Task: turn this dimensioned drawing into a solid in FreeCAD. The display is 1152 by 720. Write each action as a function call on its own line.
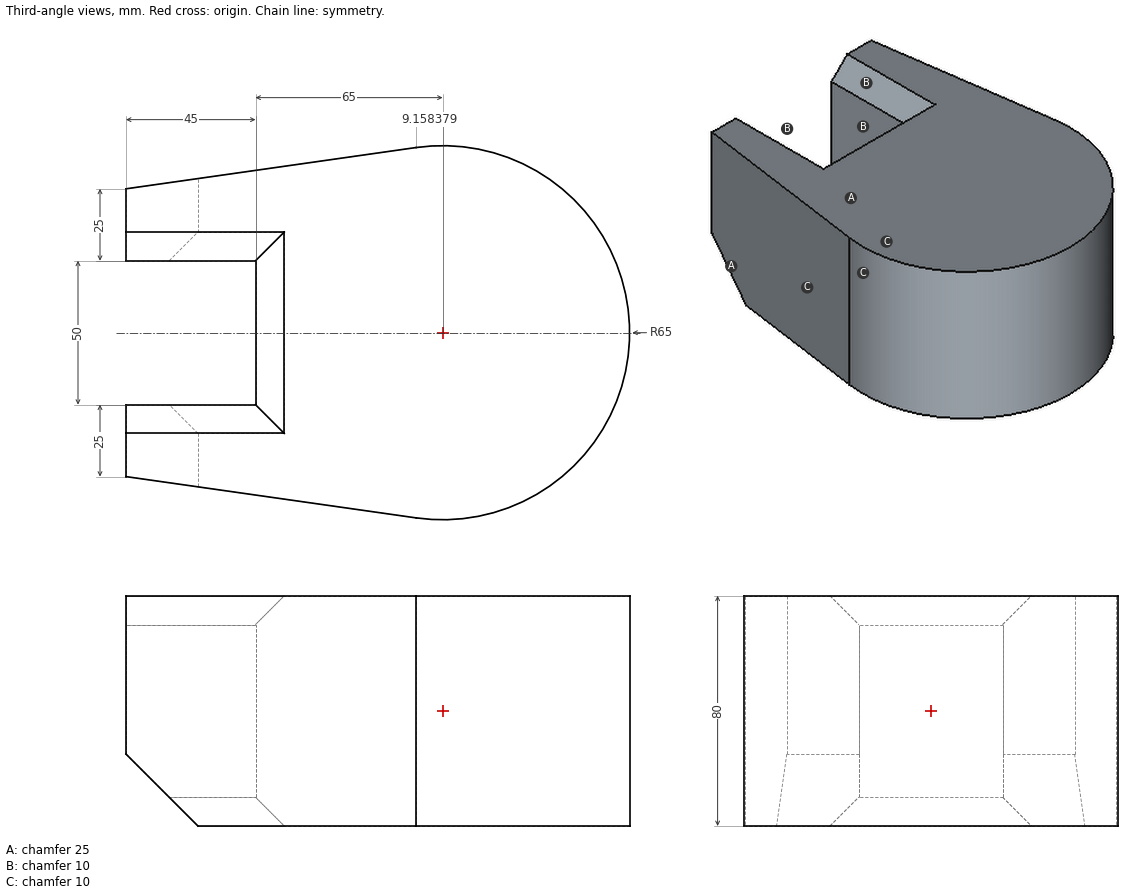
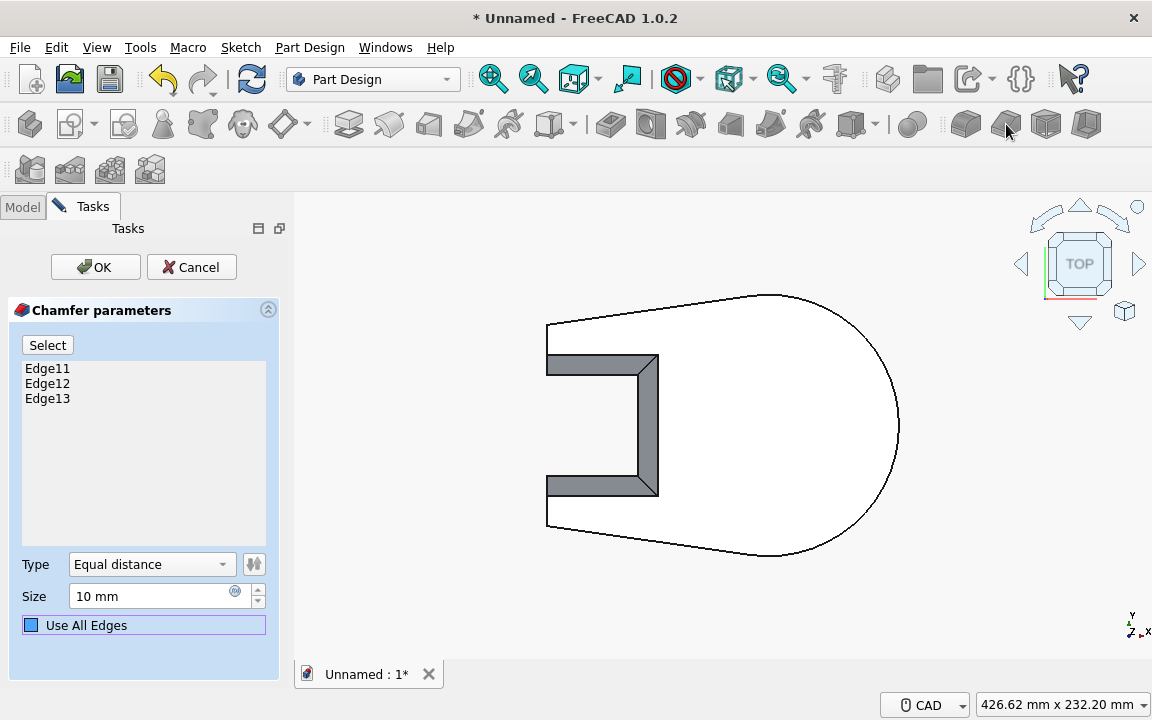
click(96, 267)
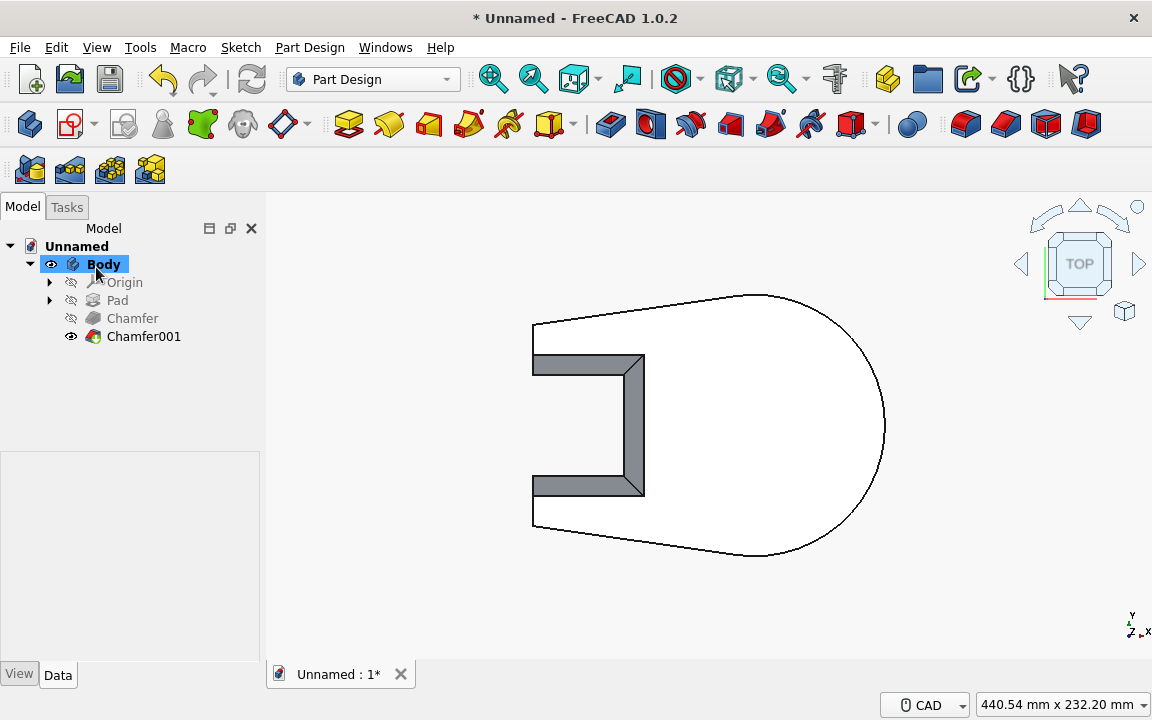
key(0)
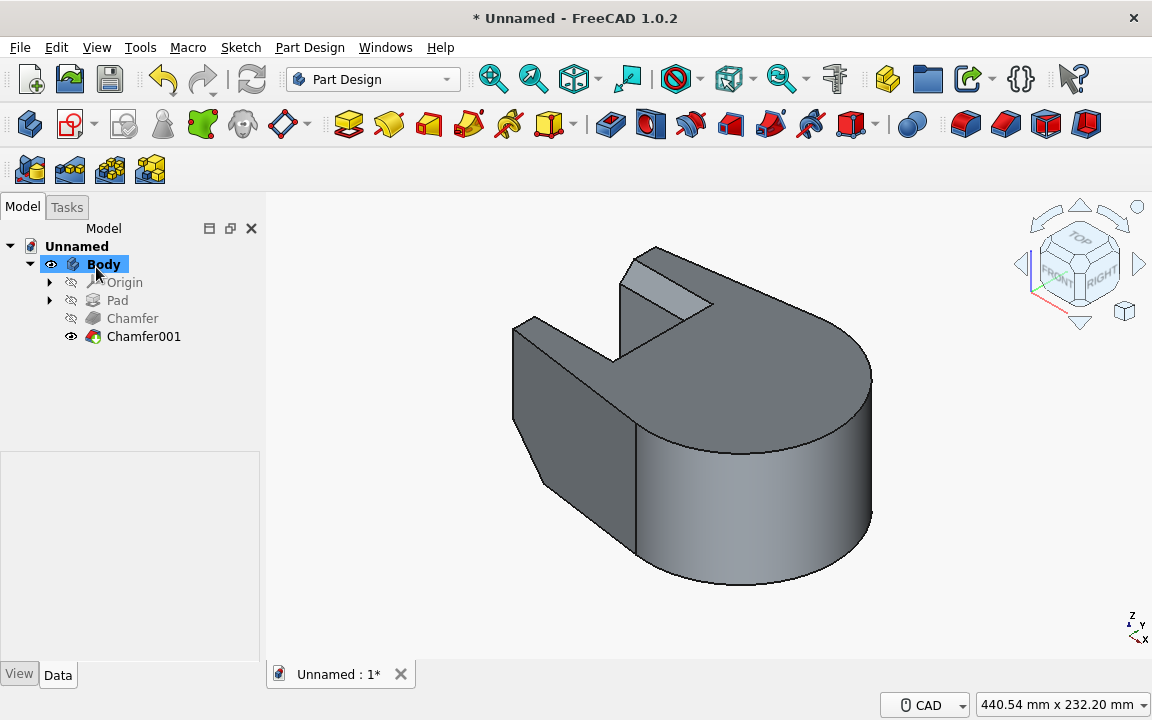
key(2)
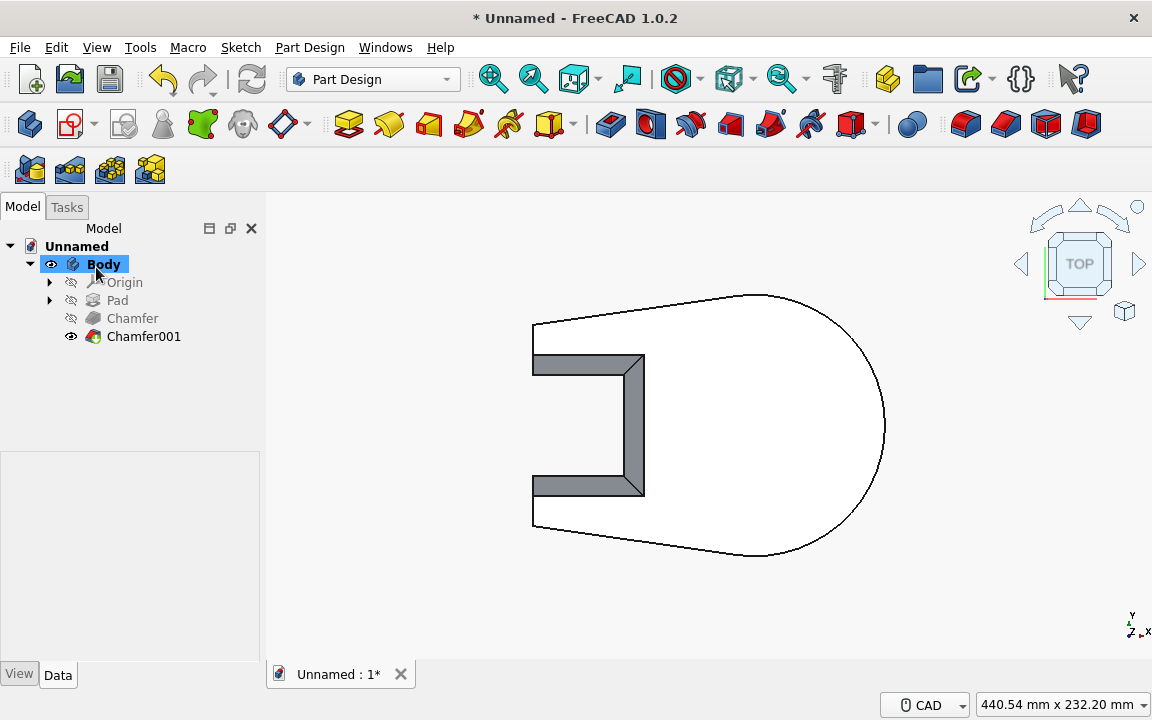
key(1)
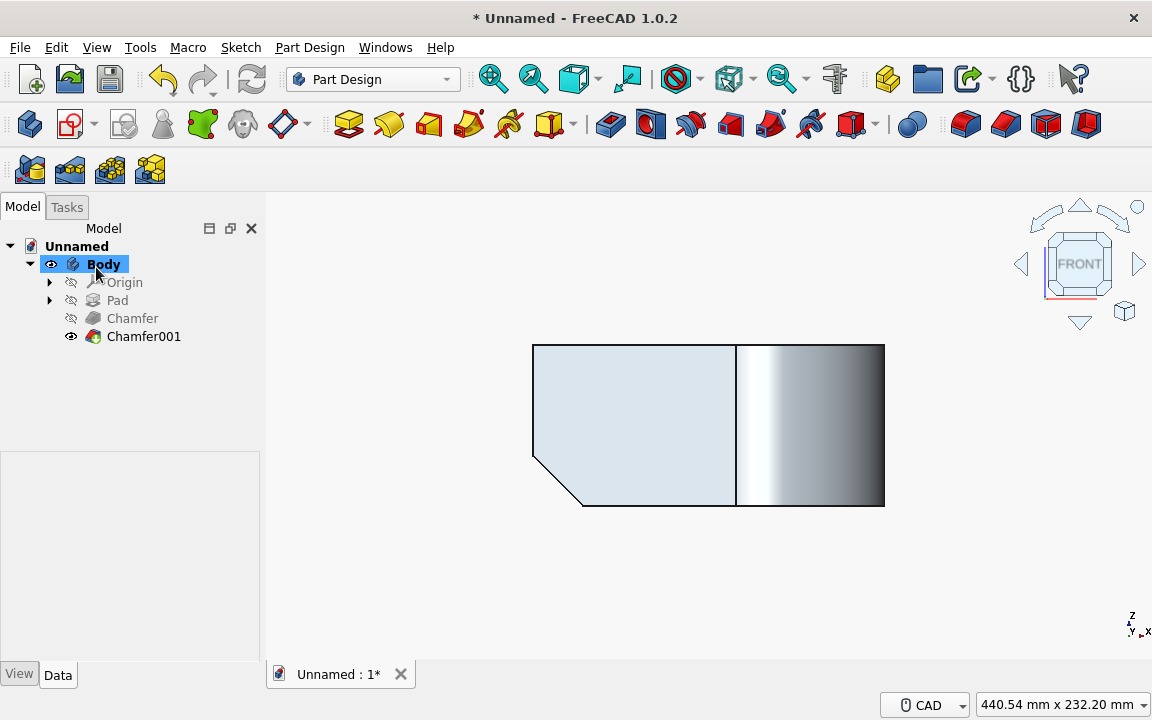
click(494, 80)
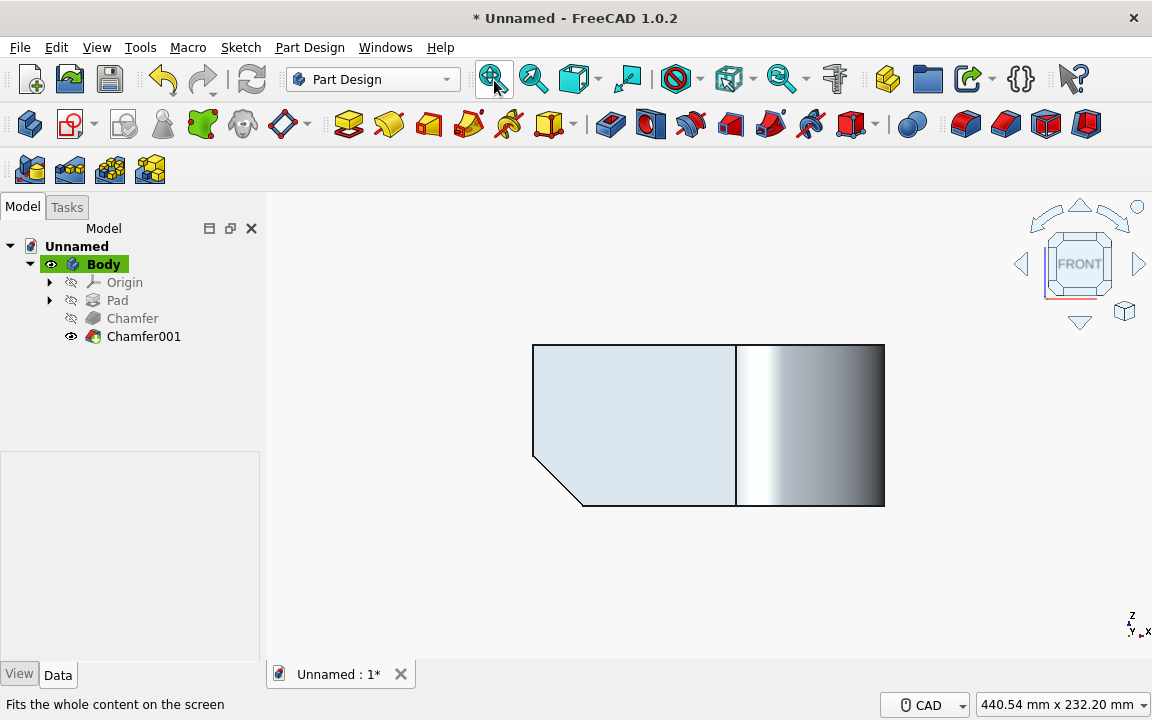
key(3)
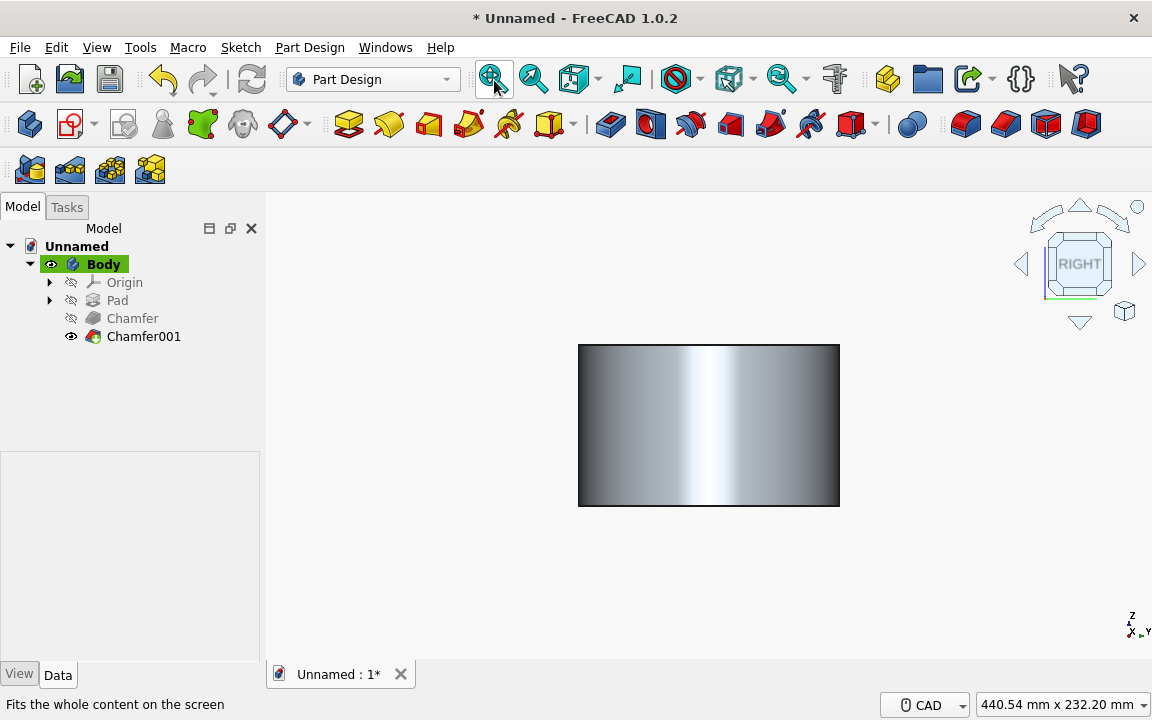
click(494, 80)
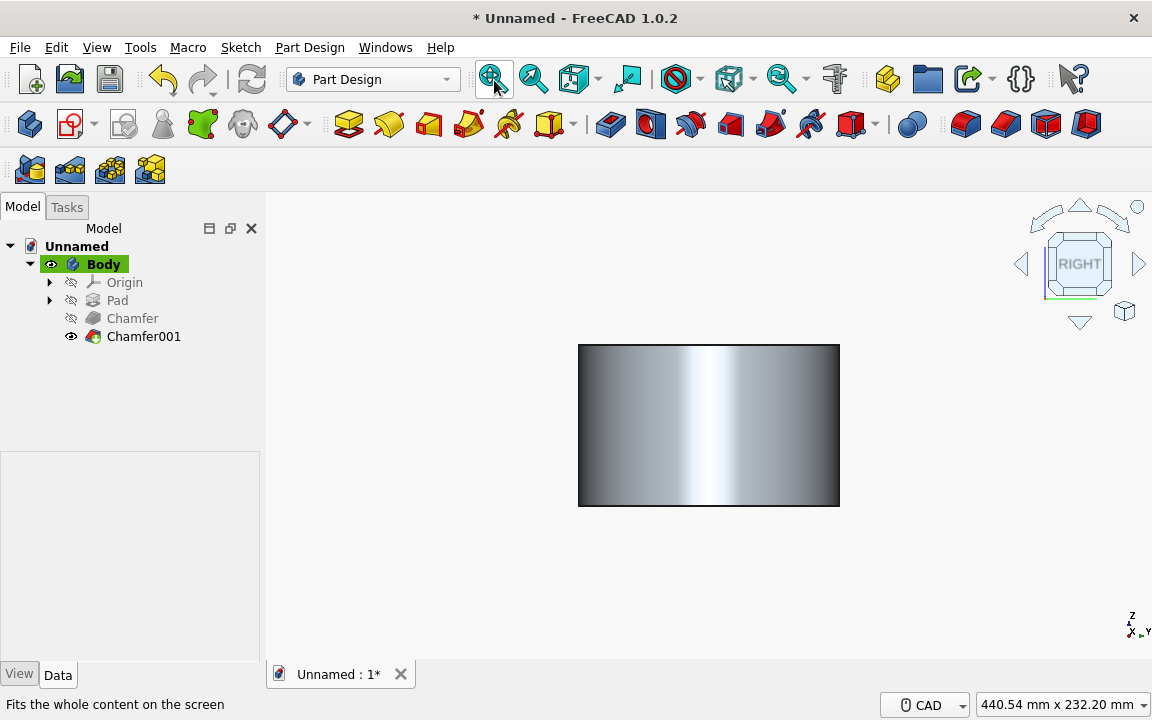
key(5)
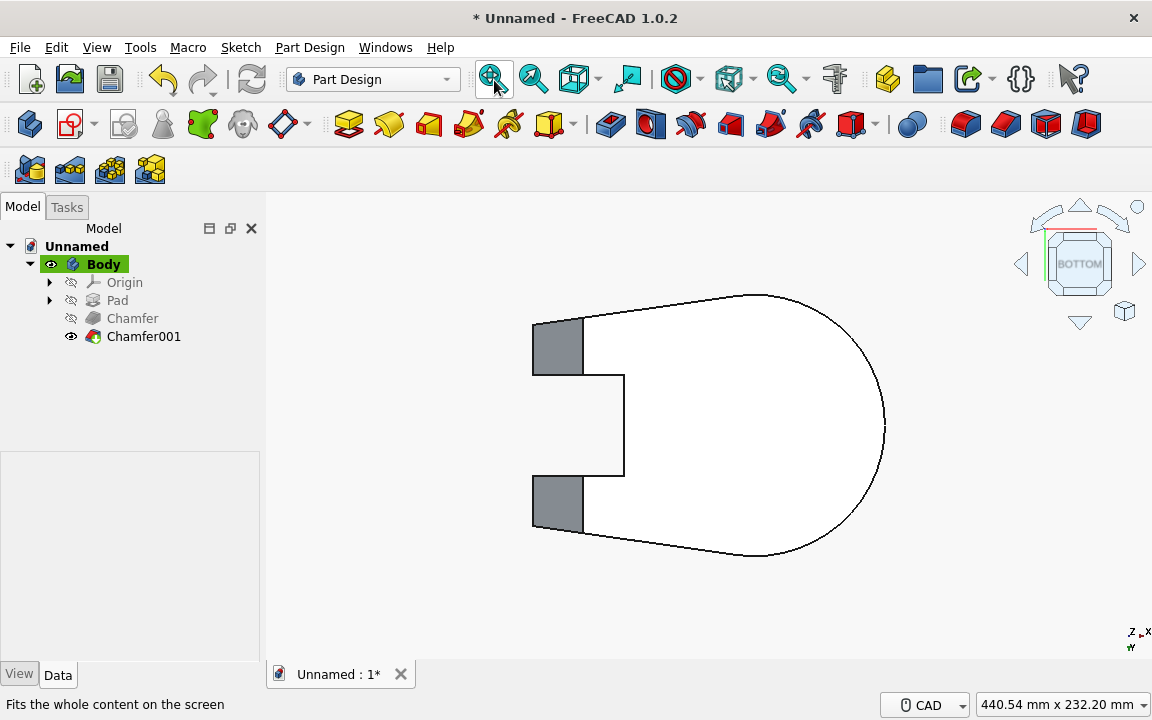
click(603, 475)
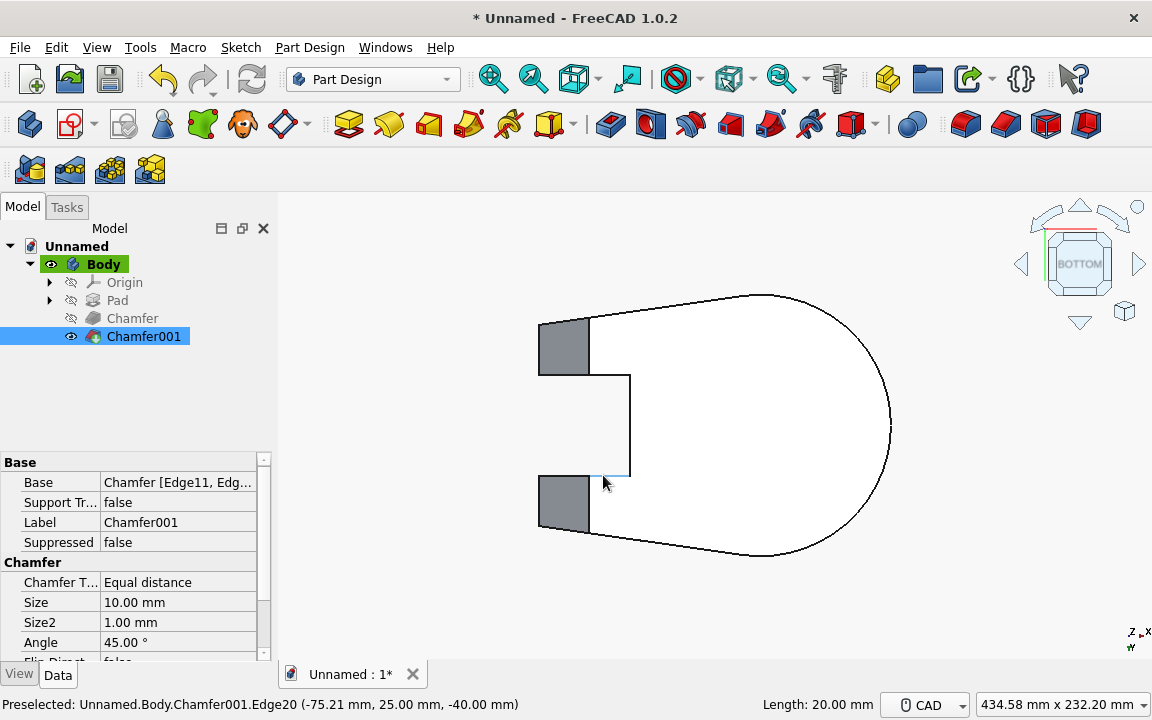
click(609, 374, ctrl)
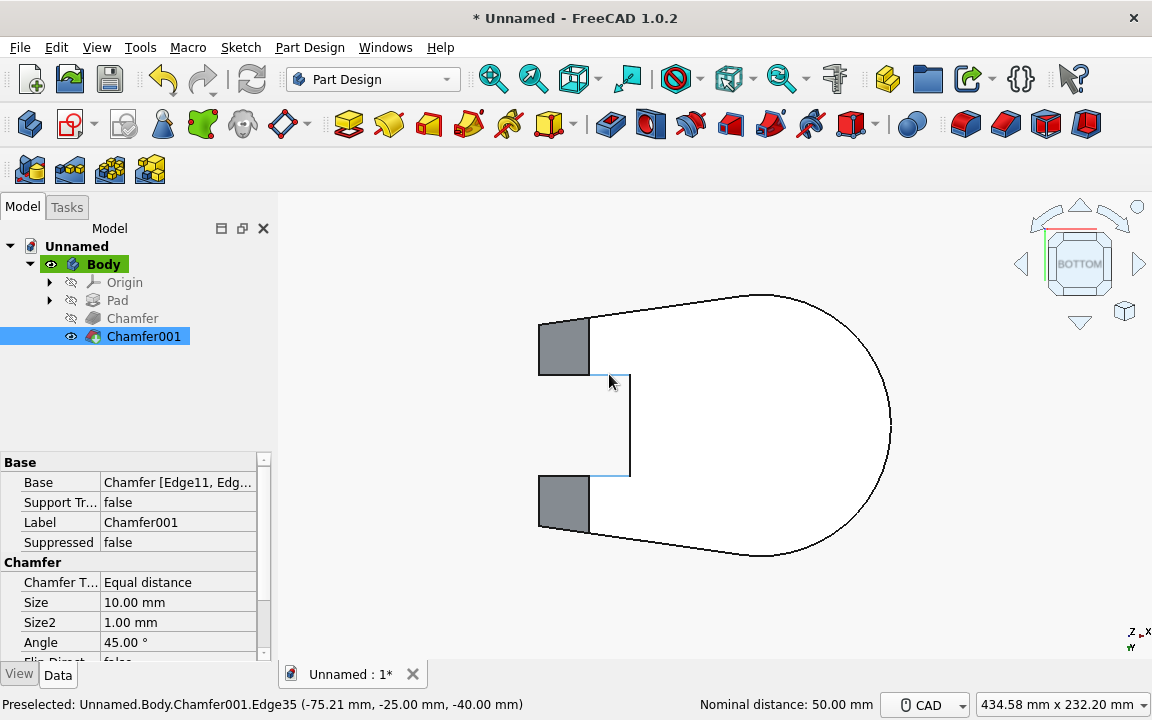
click(630, 424, ctrl)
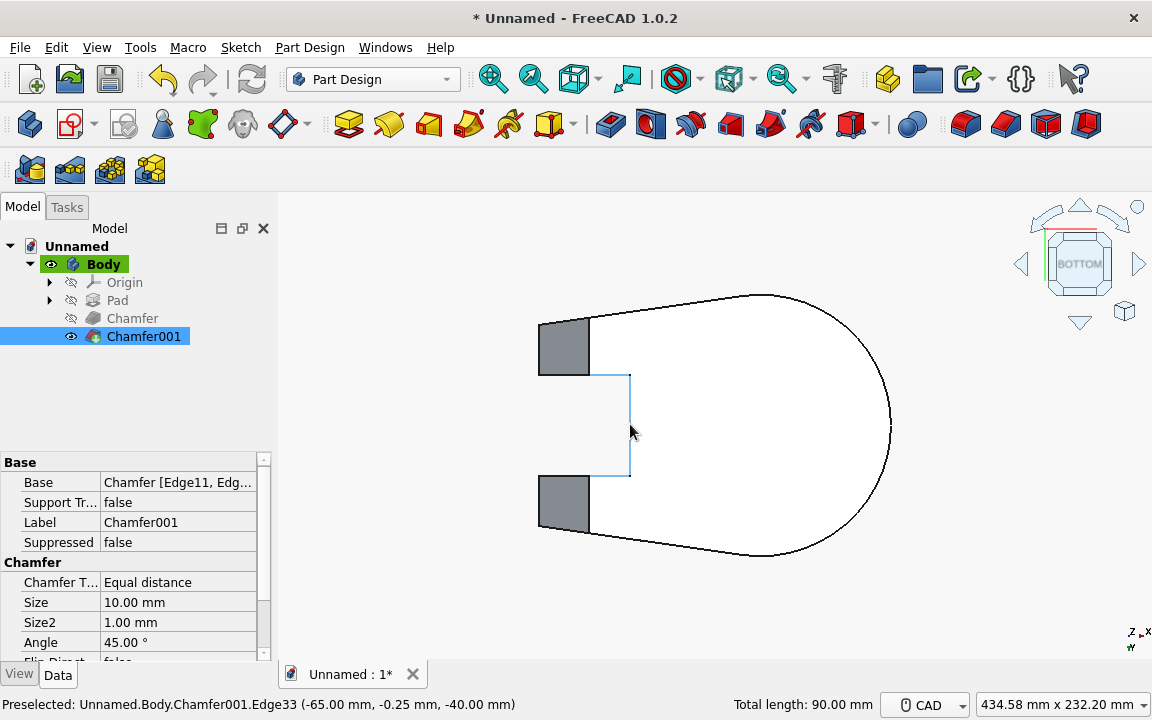
click(1006, 124)